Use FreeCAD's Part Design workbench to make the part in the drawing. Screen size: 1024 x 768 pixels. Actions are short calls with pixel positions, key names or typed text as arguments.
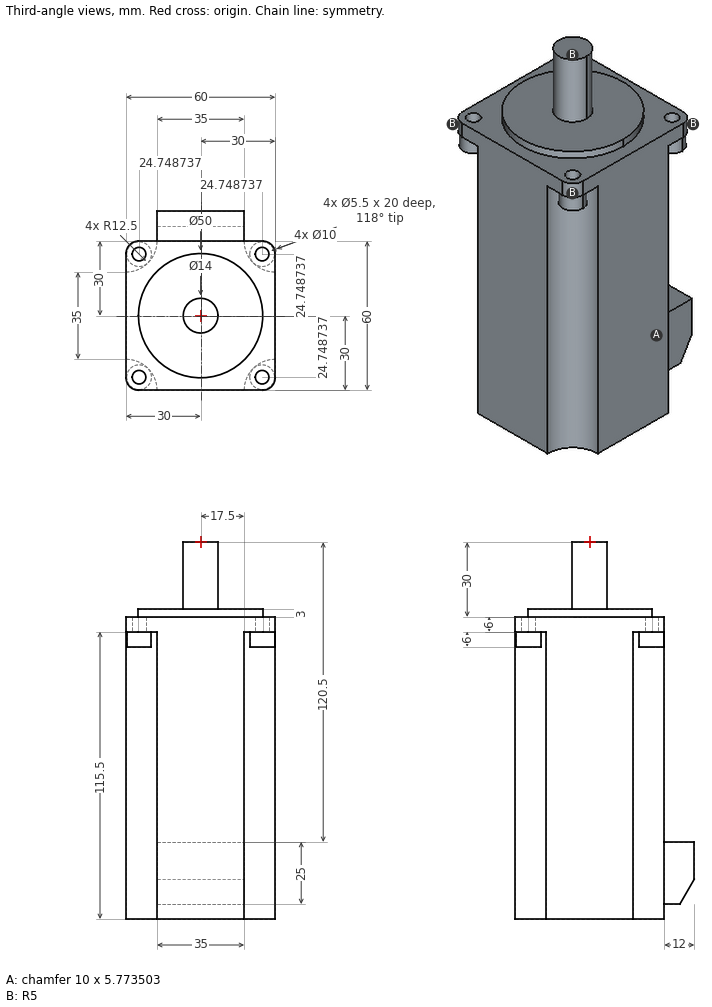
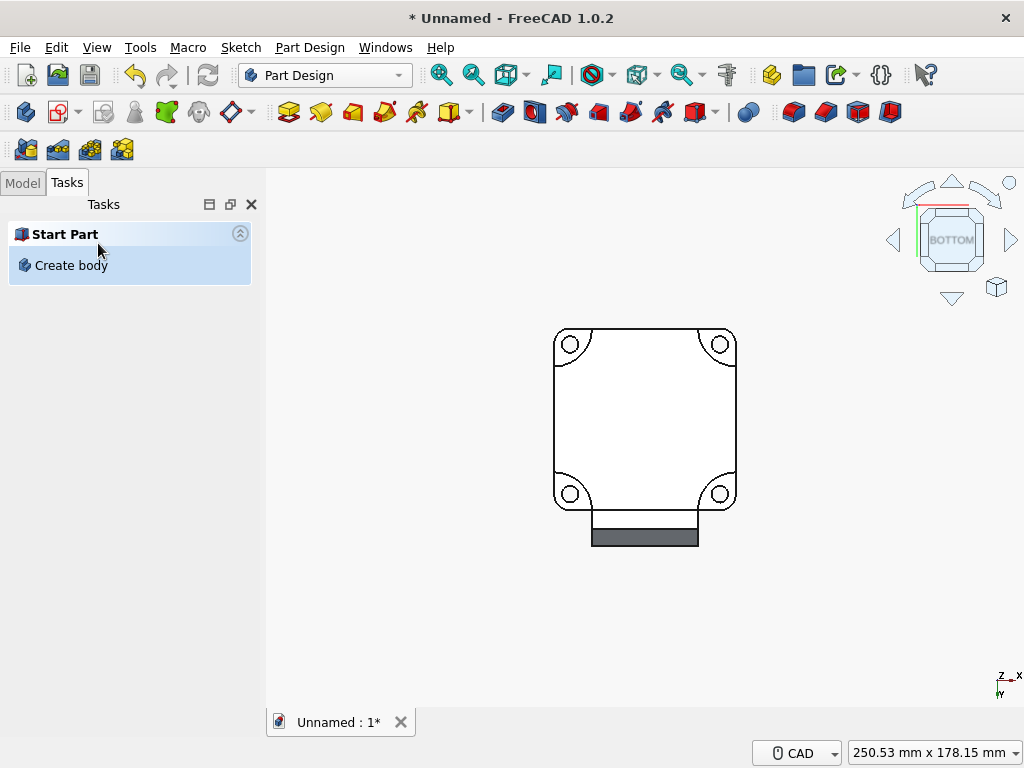
click(442, 76)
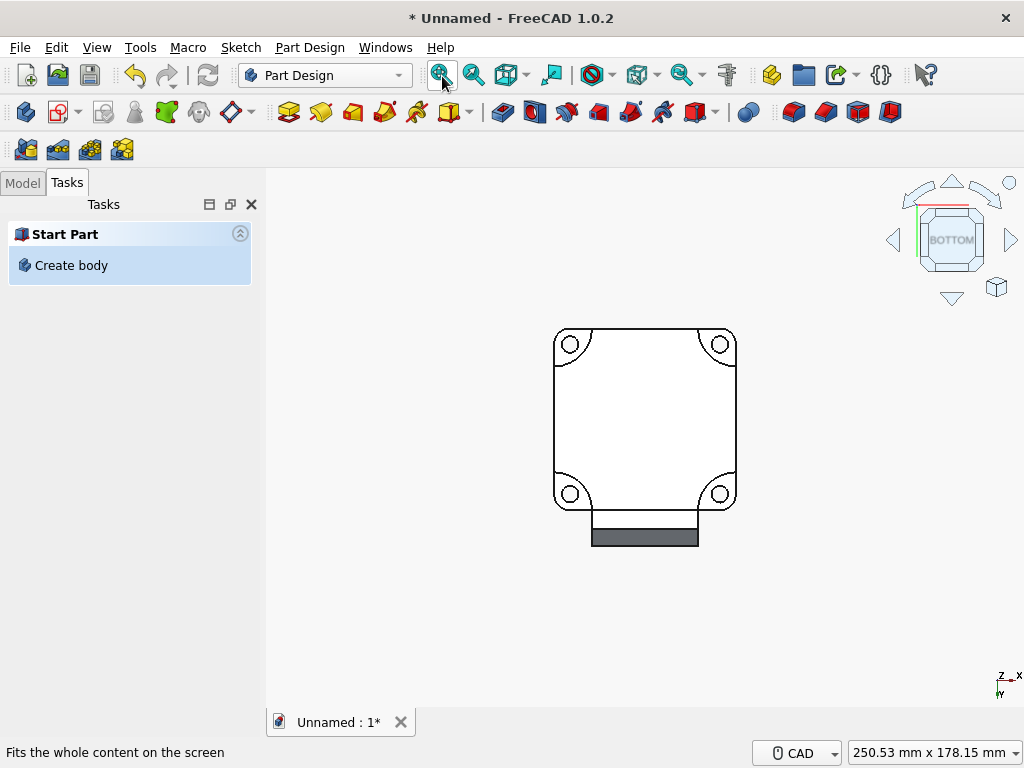
key(1)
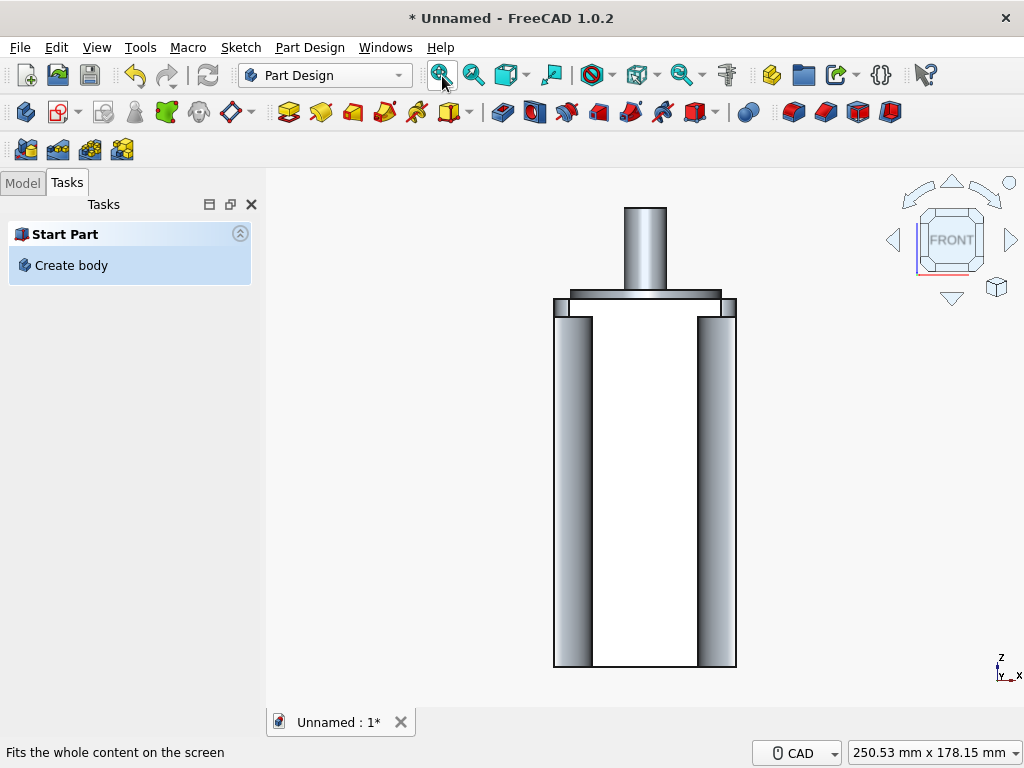
key(3)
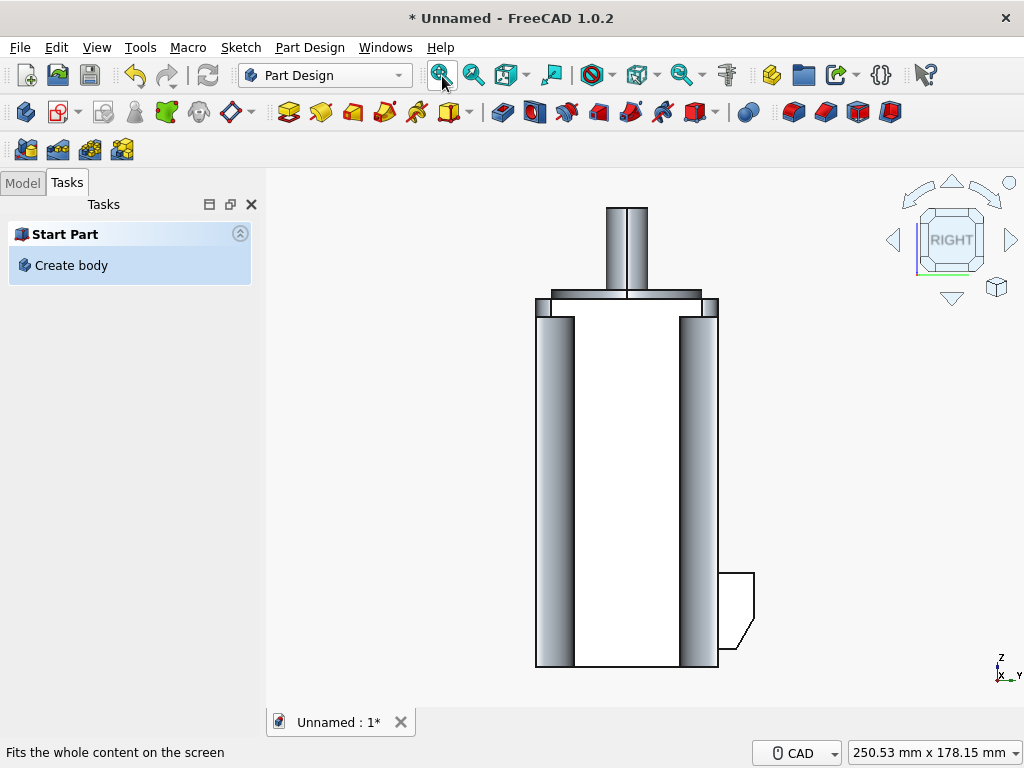
click(23, 182)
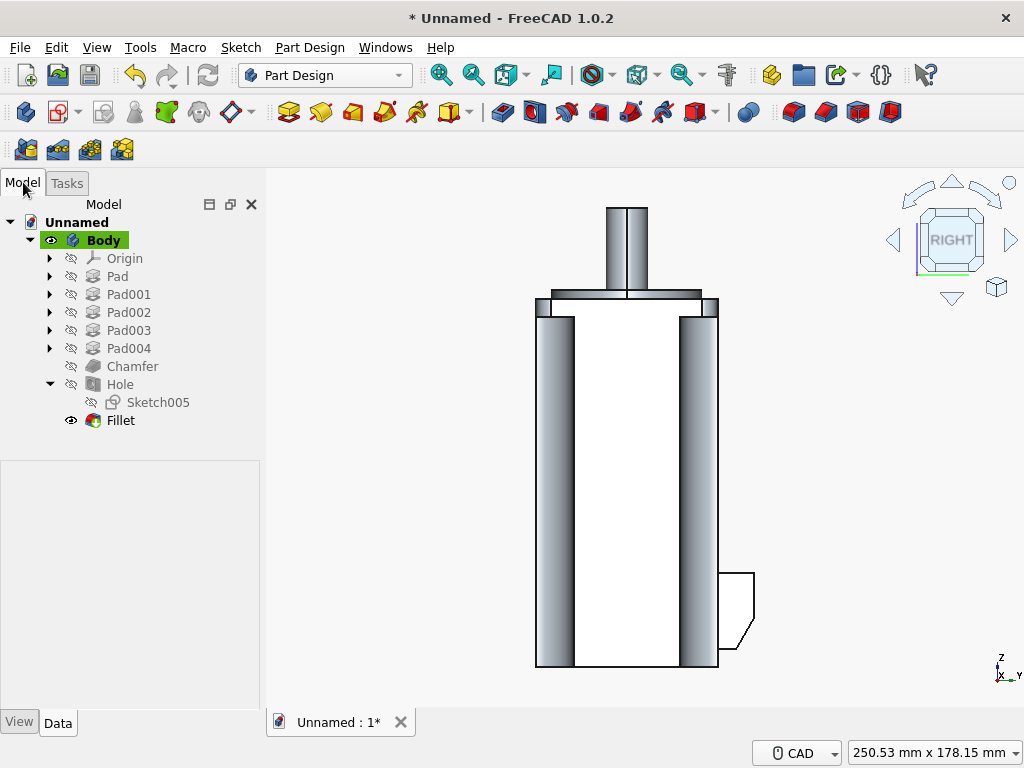
click(50, 258)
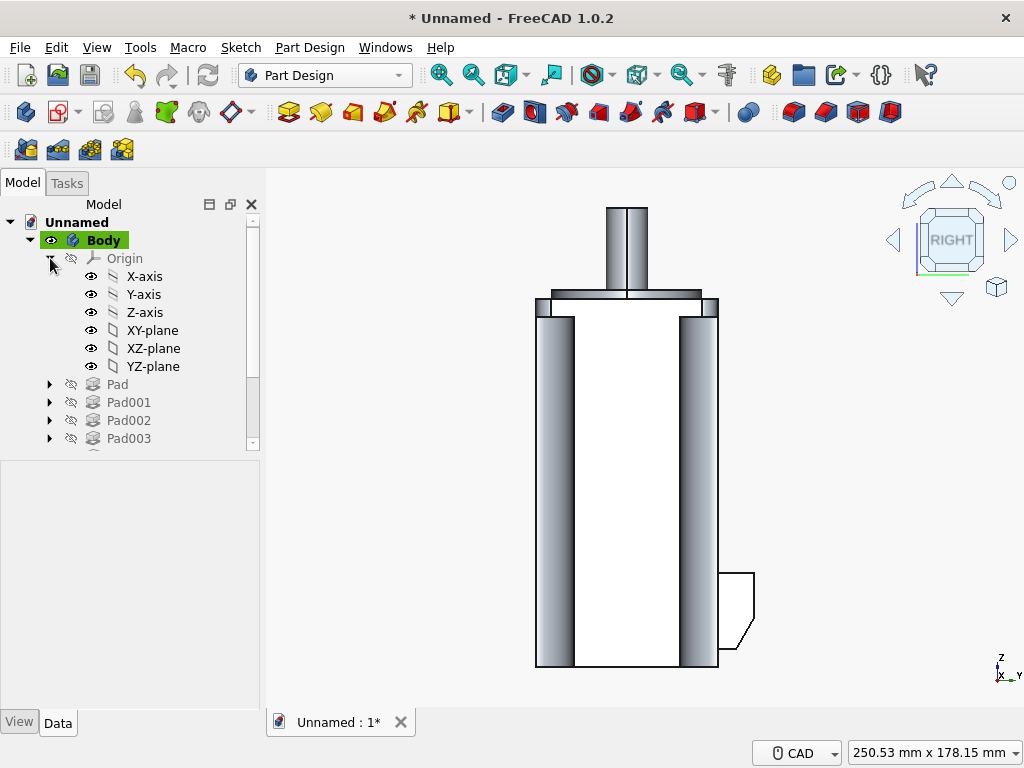
click(136, 330)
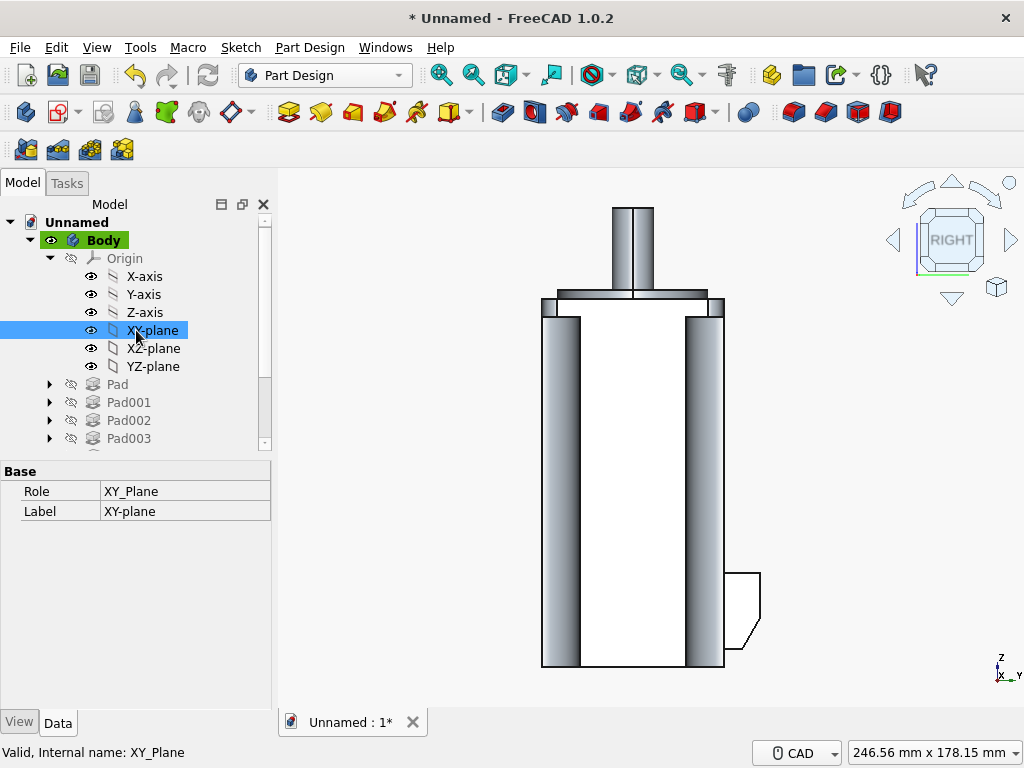
click(232, 112)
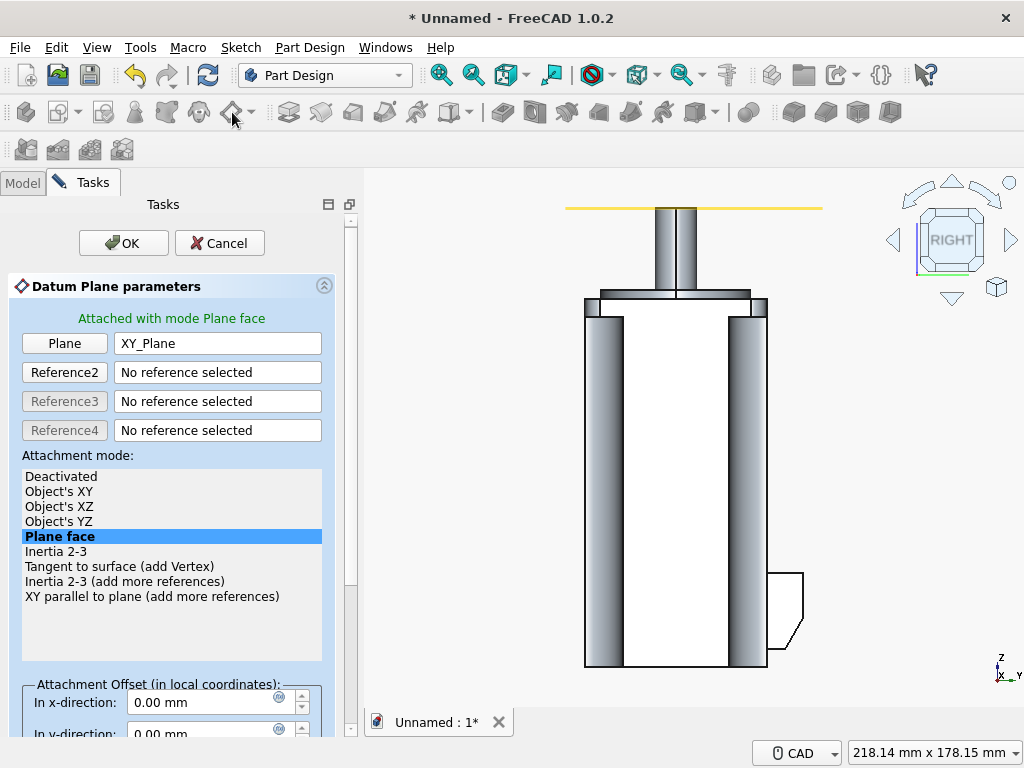
scroll(351, 475, down, 2)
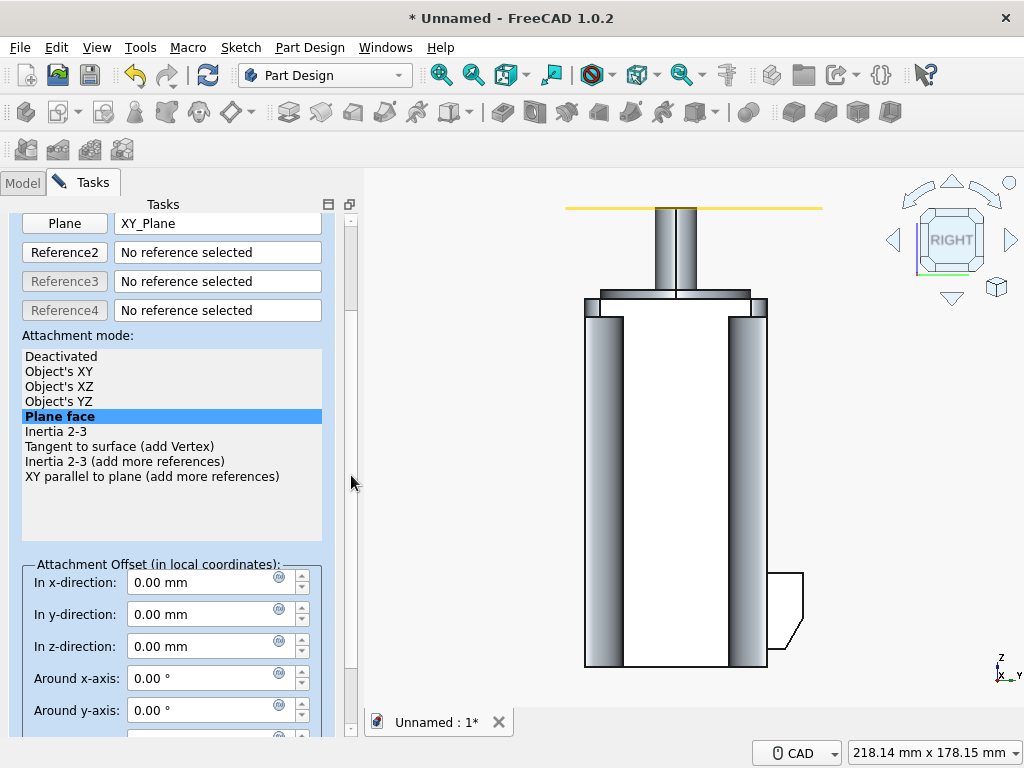
triple_click(210, 646)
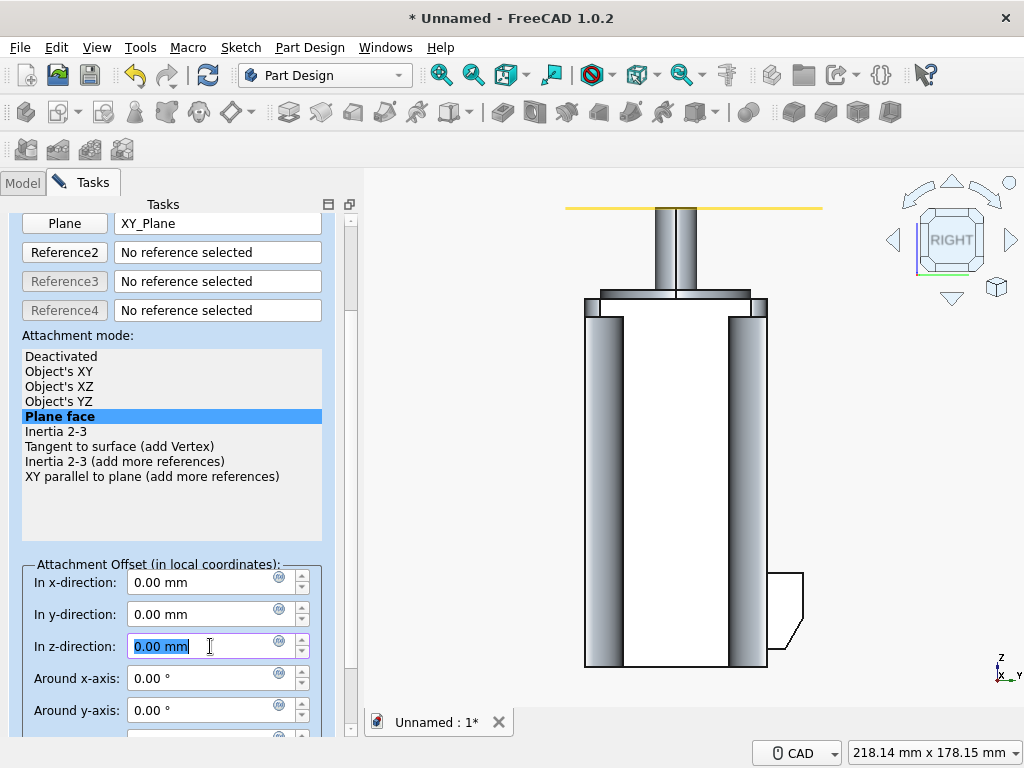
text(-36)
key(Tab)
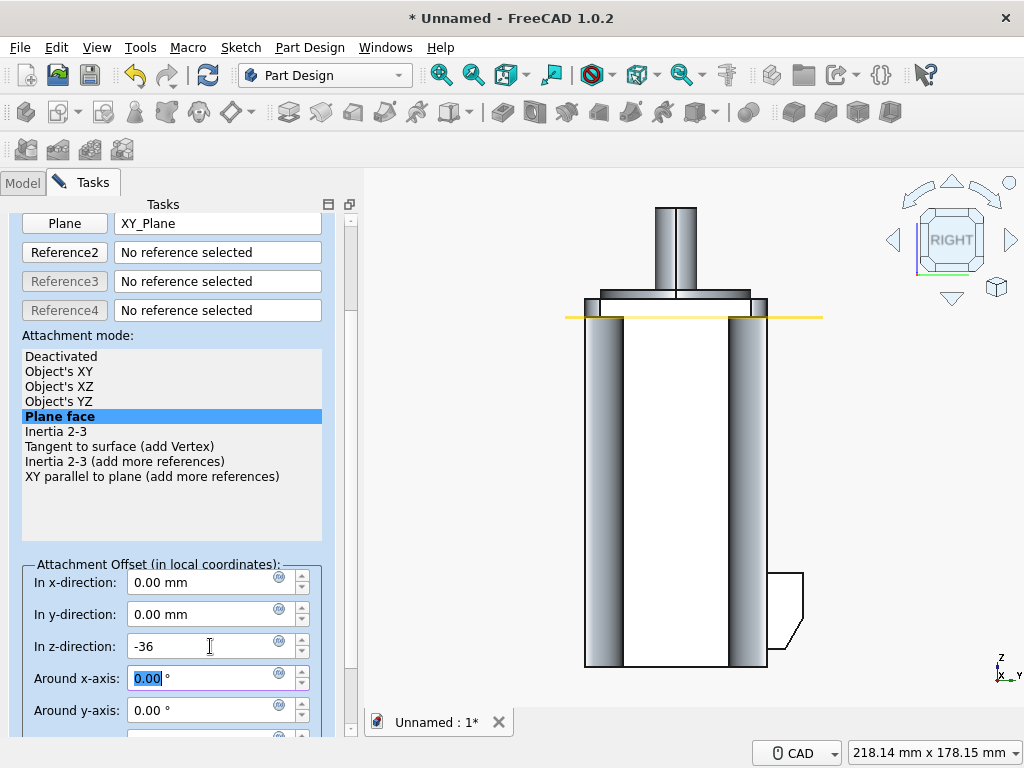
scroll(351, 475, up, 3)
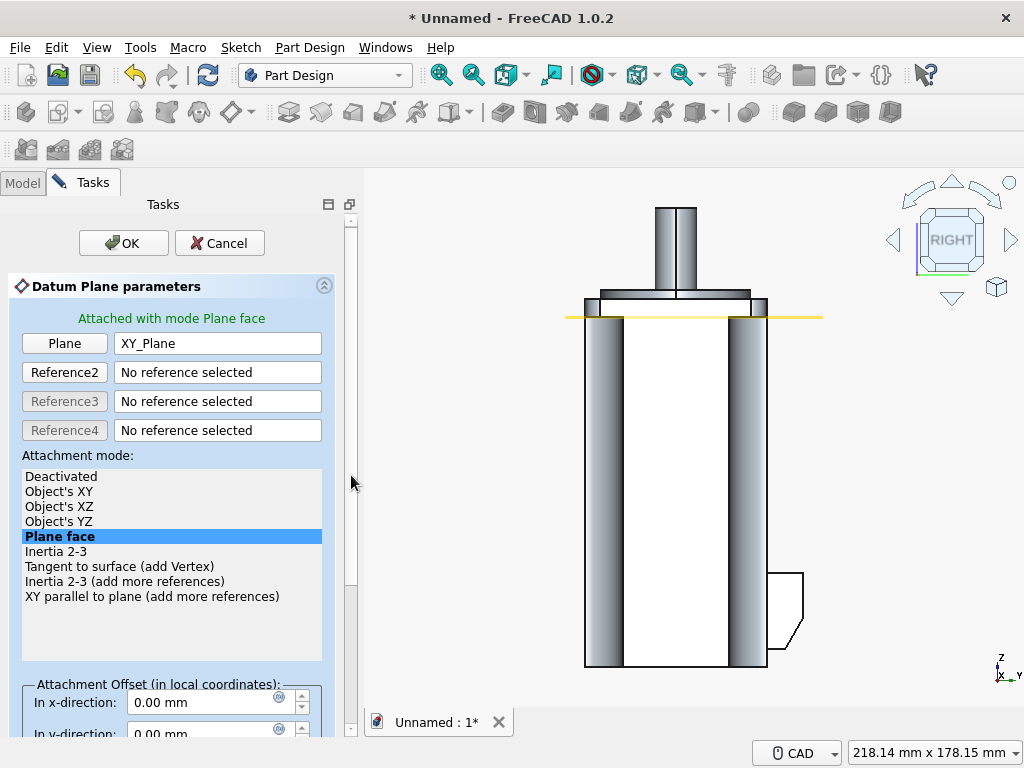
click(124, 243)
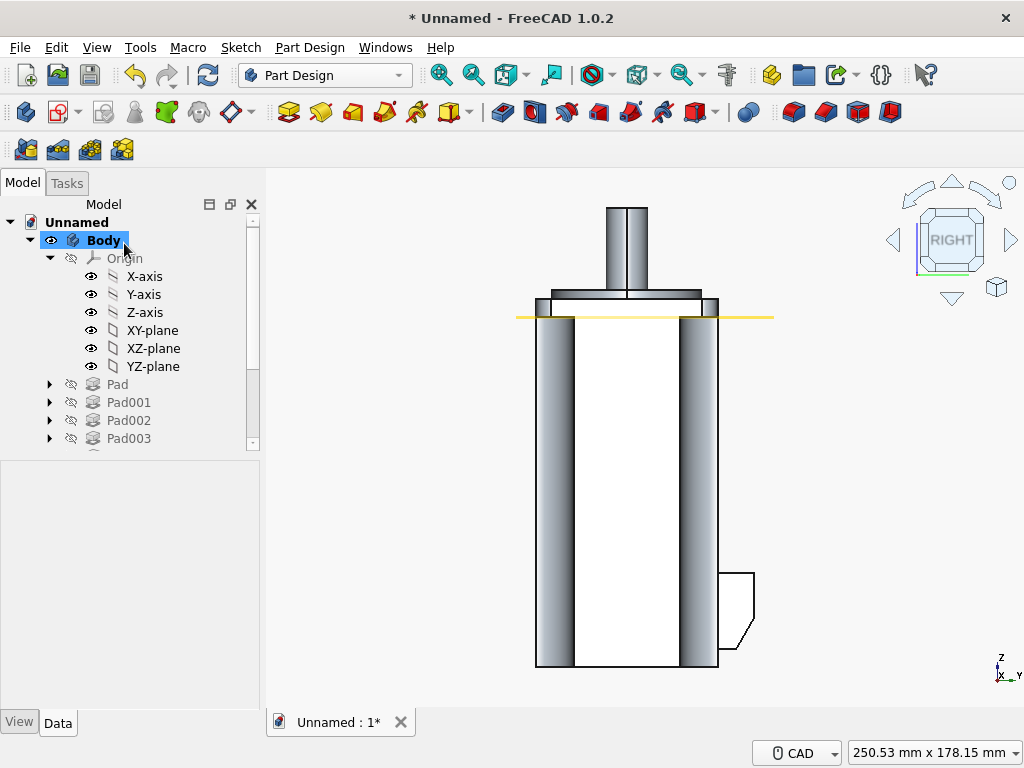
scroll(100, 326, down, 3)